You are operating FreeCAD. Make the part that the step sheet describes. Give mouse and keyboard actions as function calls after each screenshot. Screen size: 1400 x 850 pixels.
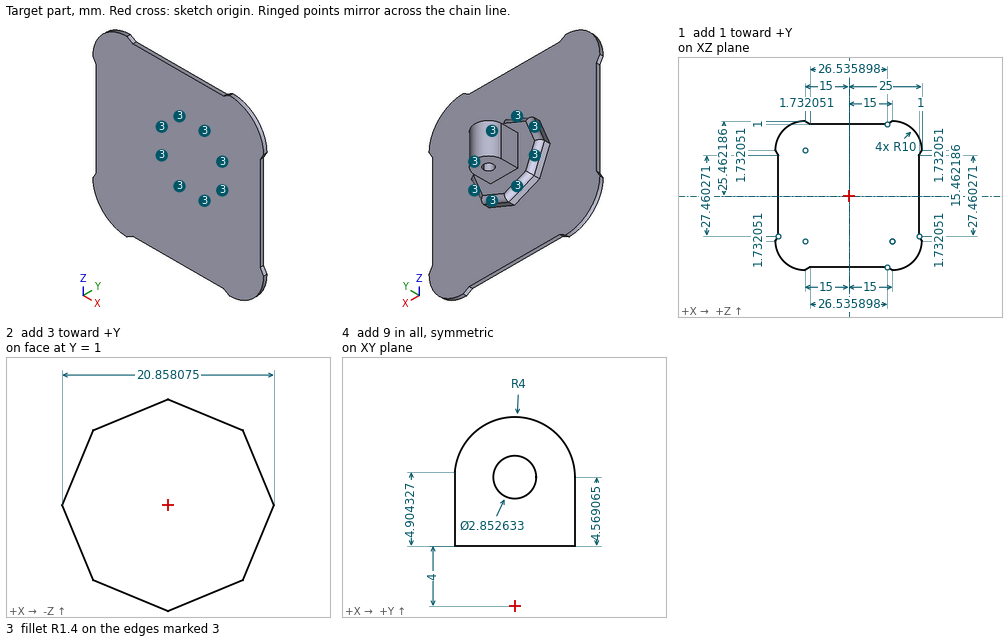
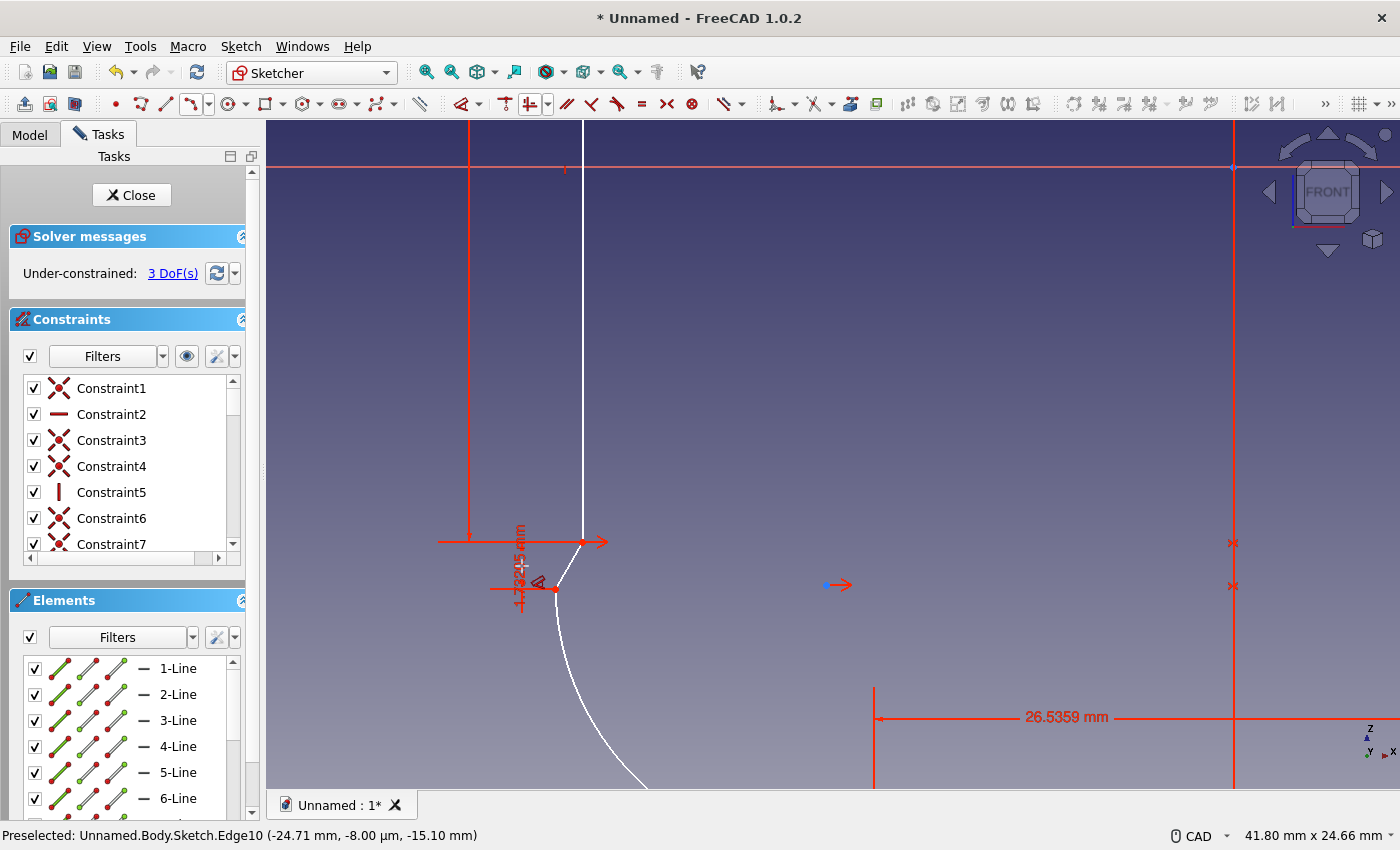
scroll(562, 578, down, 6)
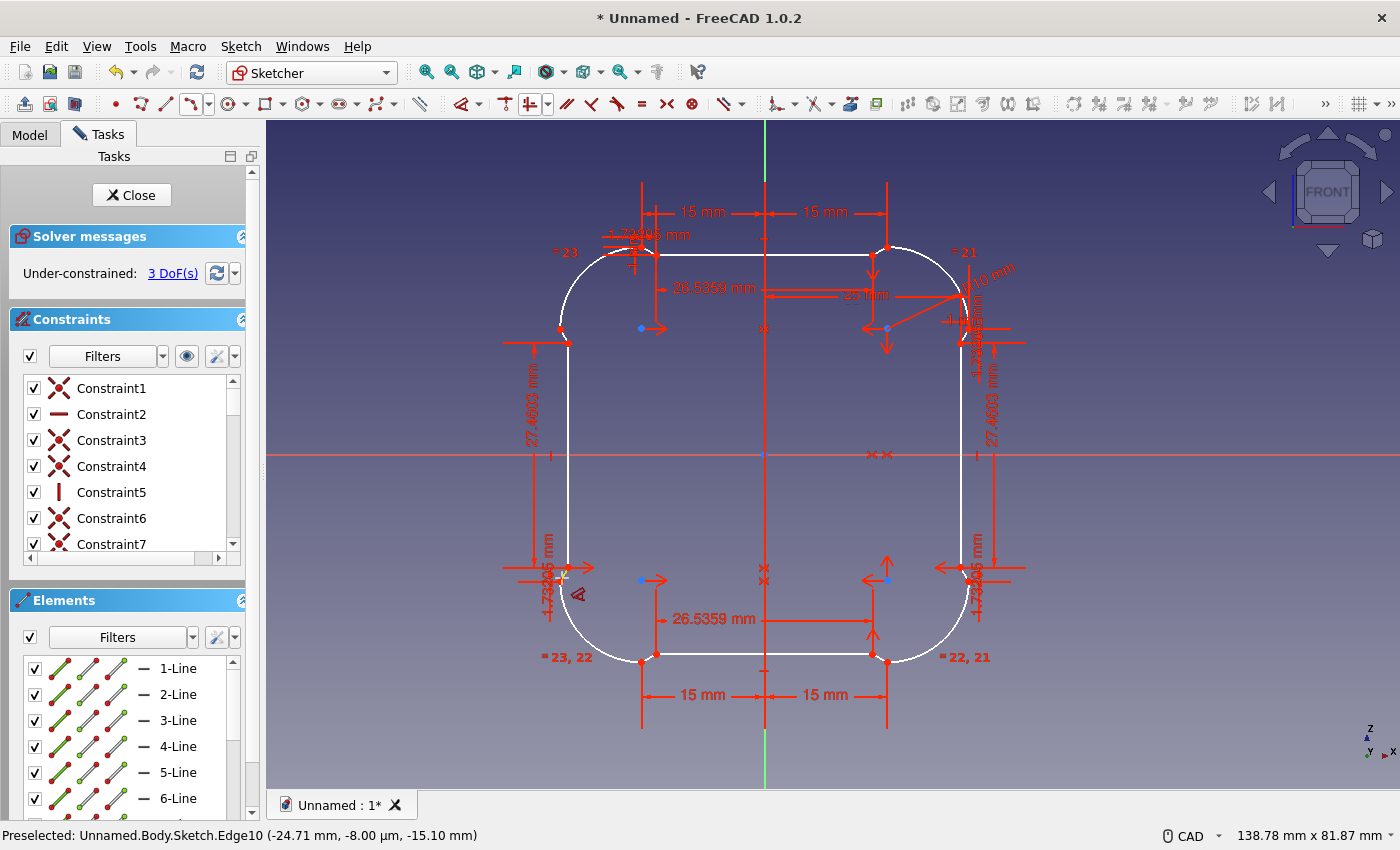
scroll(566, 339, up, 6)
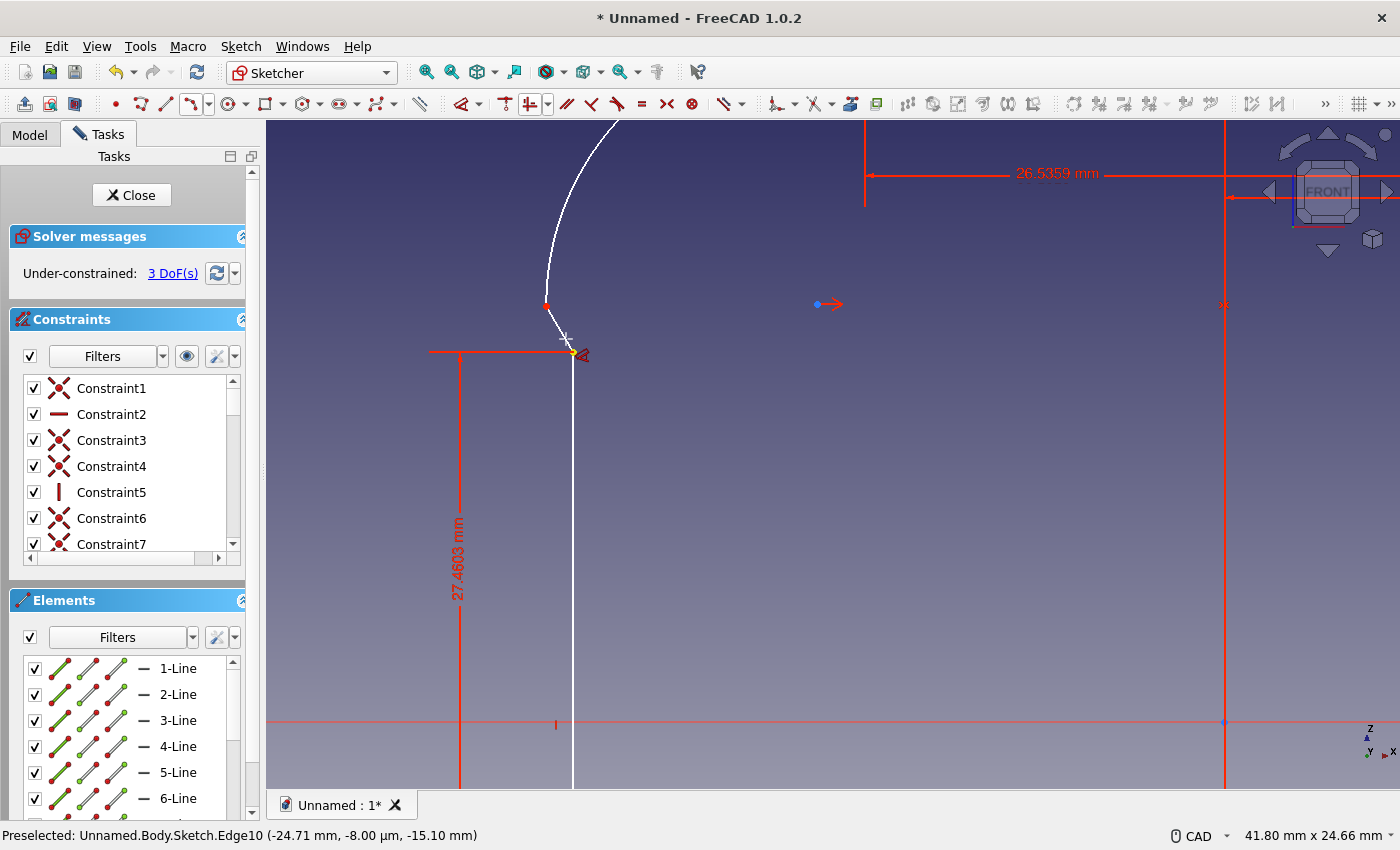
click(565, 339)
click(512, 330)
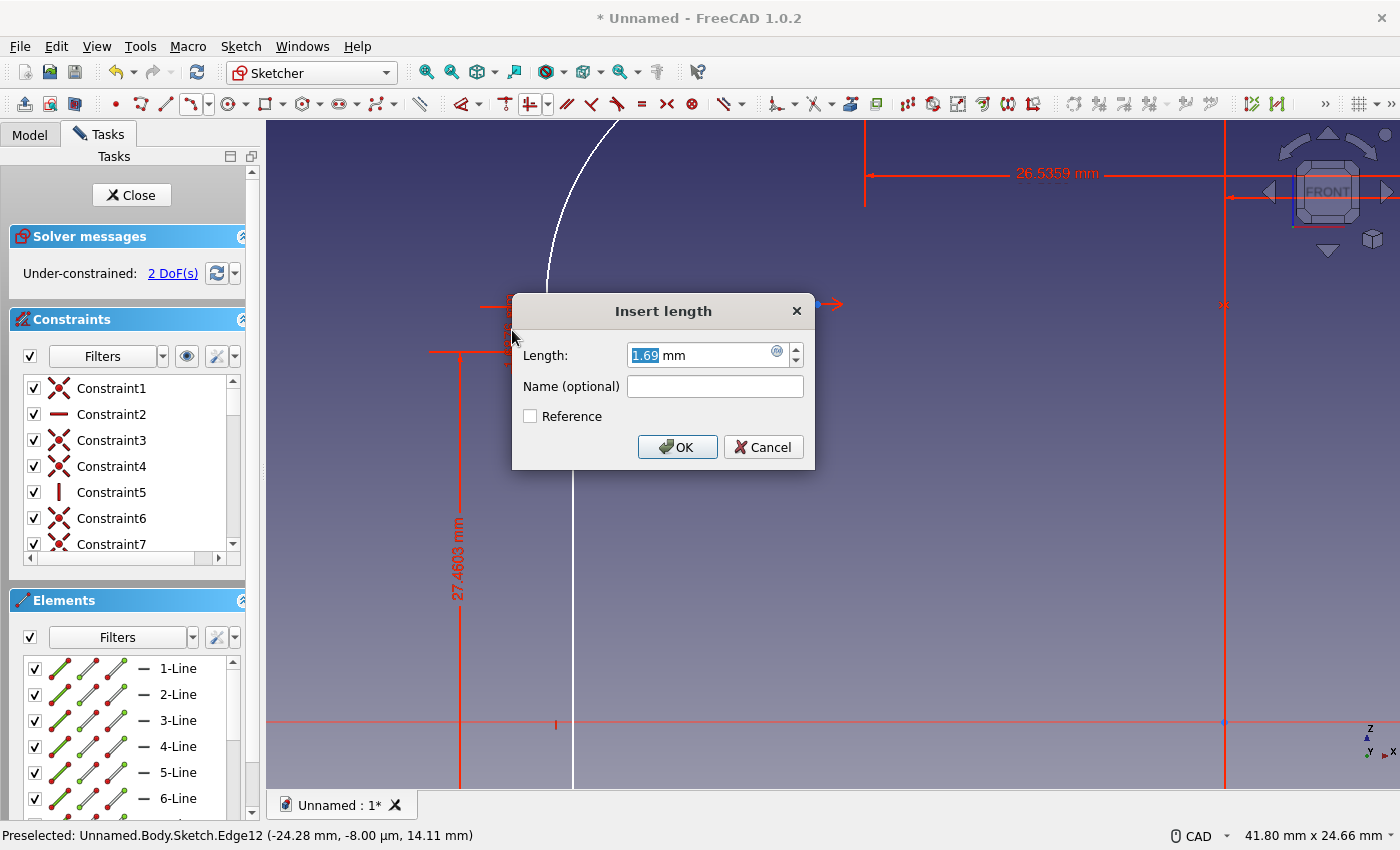
text(1.732051)
key(Return)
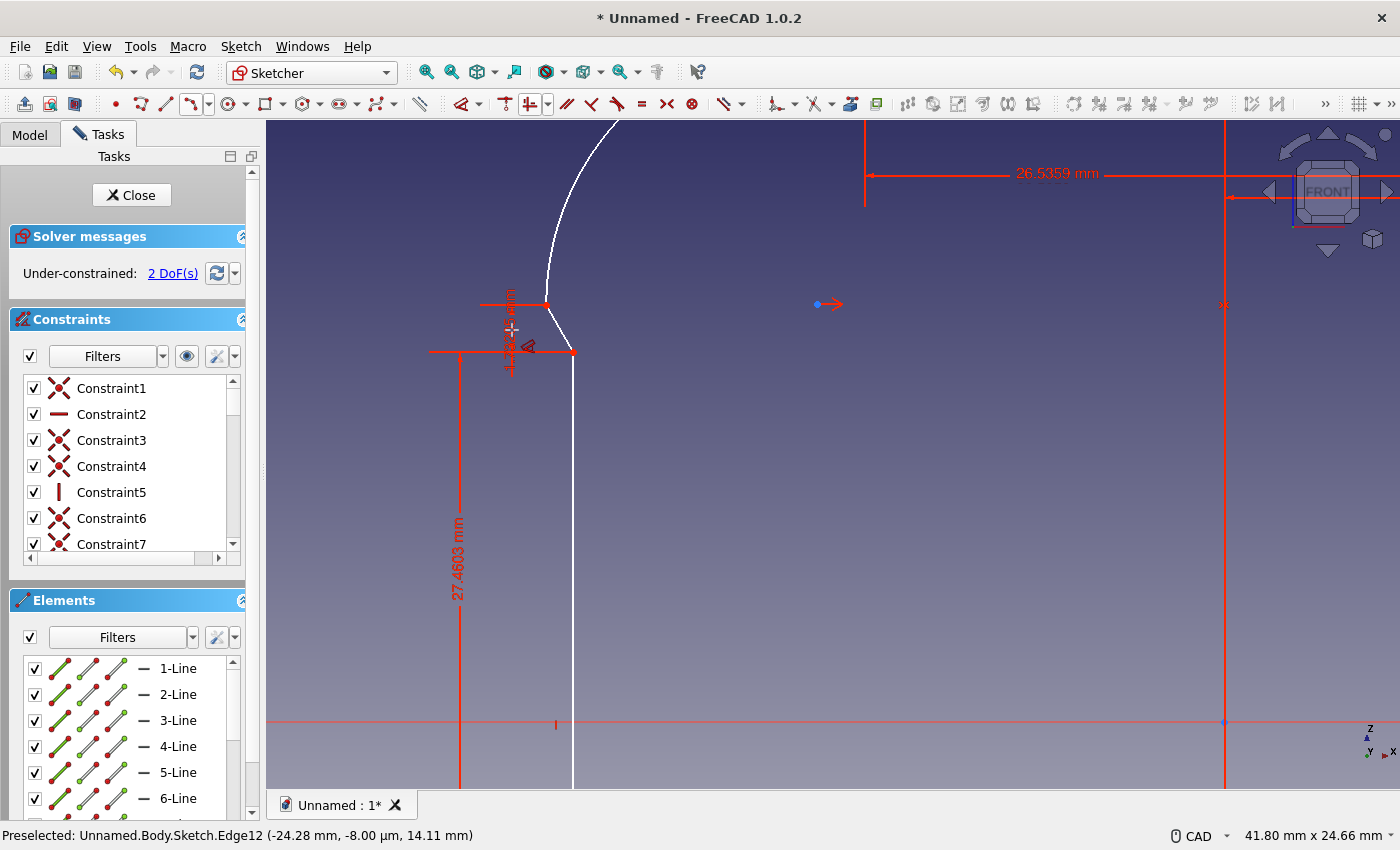
scroll(566, 339, down, 6)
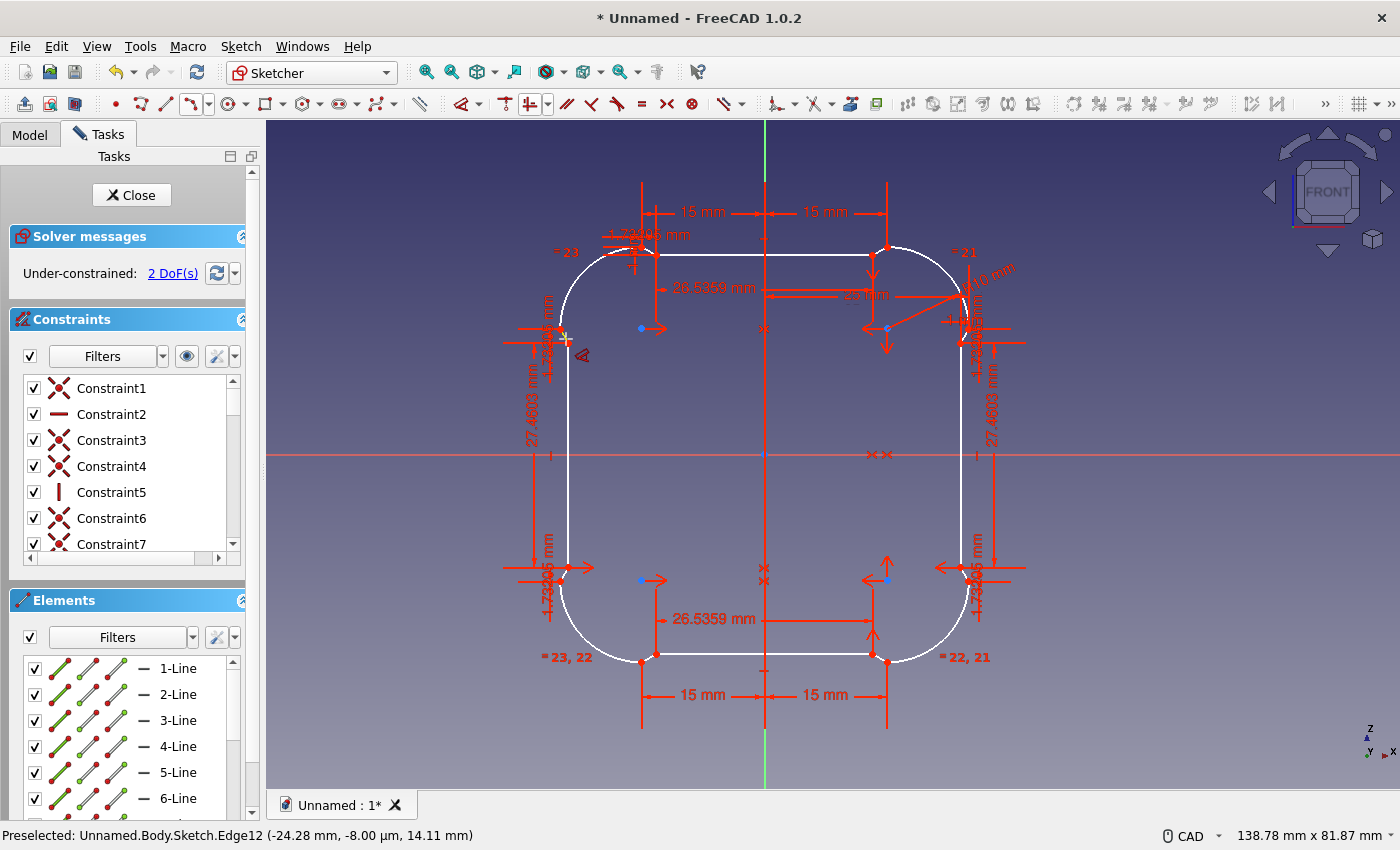
click(642, 247)
click(608, 303)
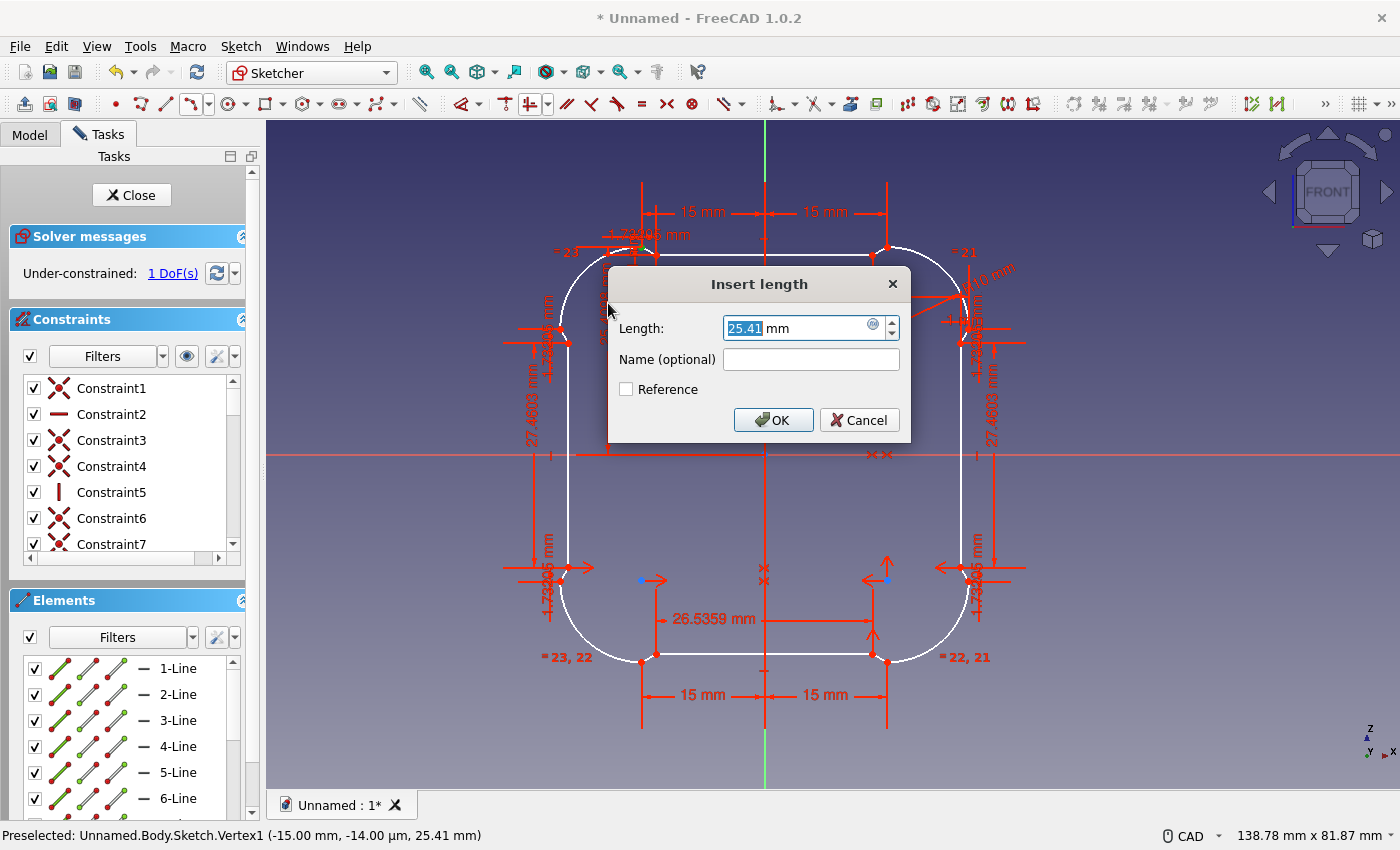
text(25.462186)
key(Return)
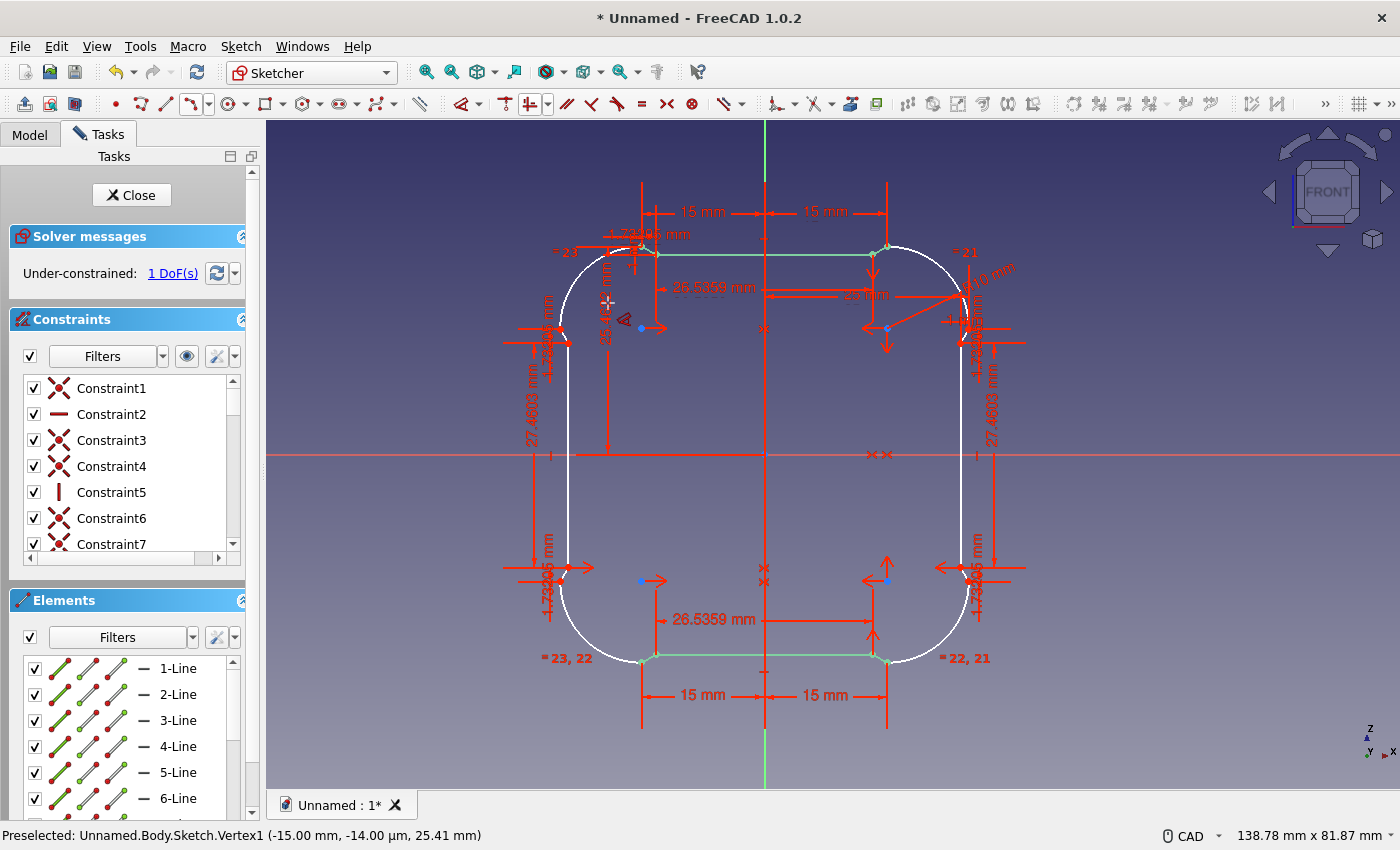
click(969, 329)
click(1003, 363)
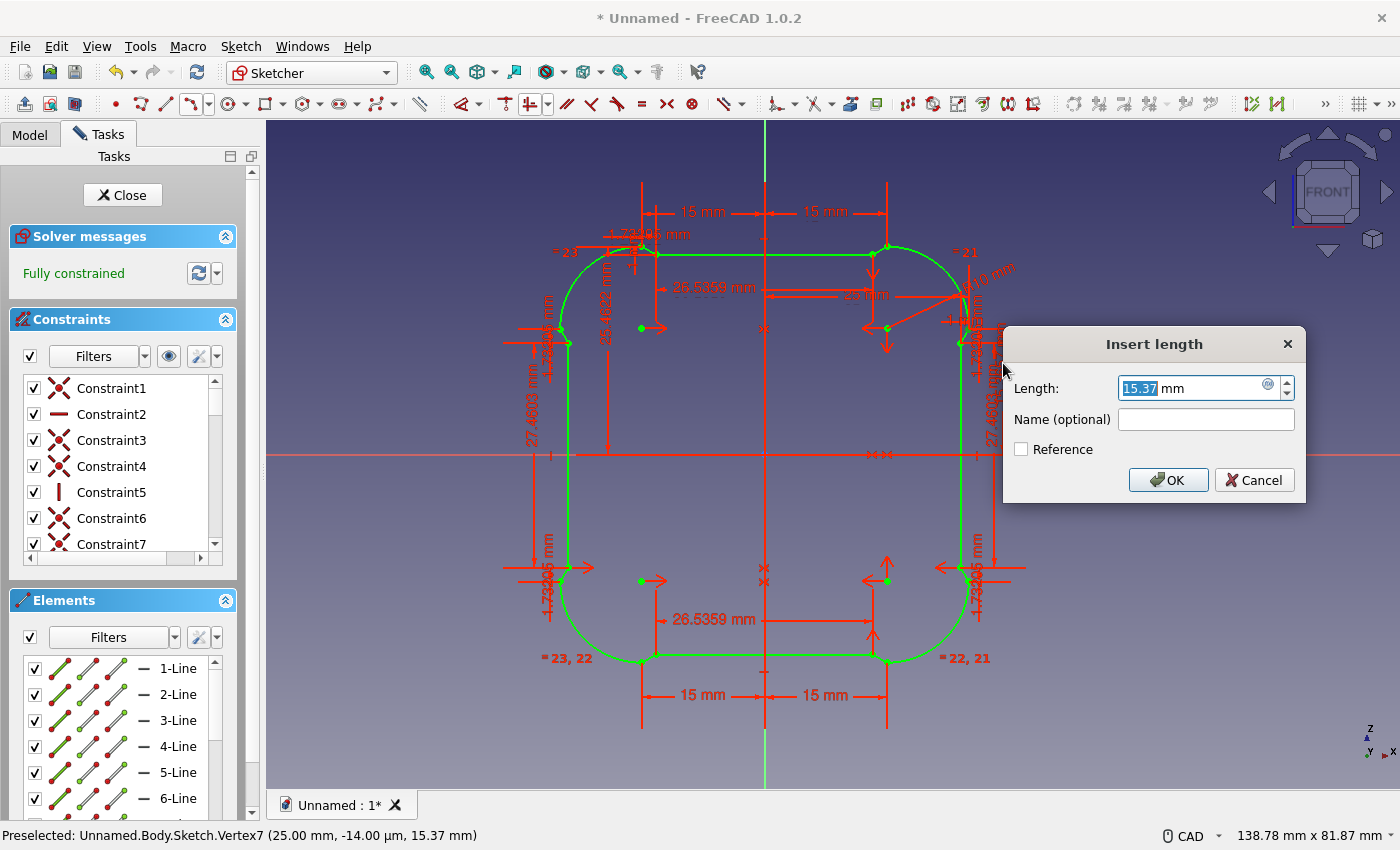
text(15.462186)
key(Return)
key(Escape)